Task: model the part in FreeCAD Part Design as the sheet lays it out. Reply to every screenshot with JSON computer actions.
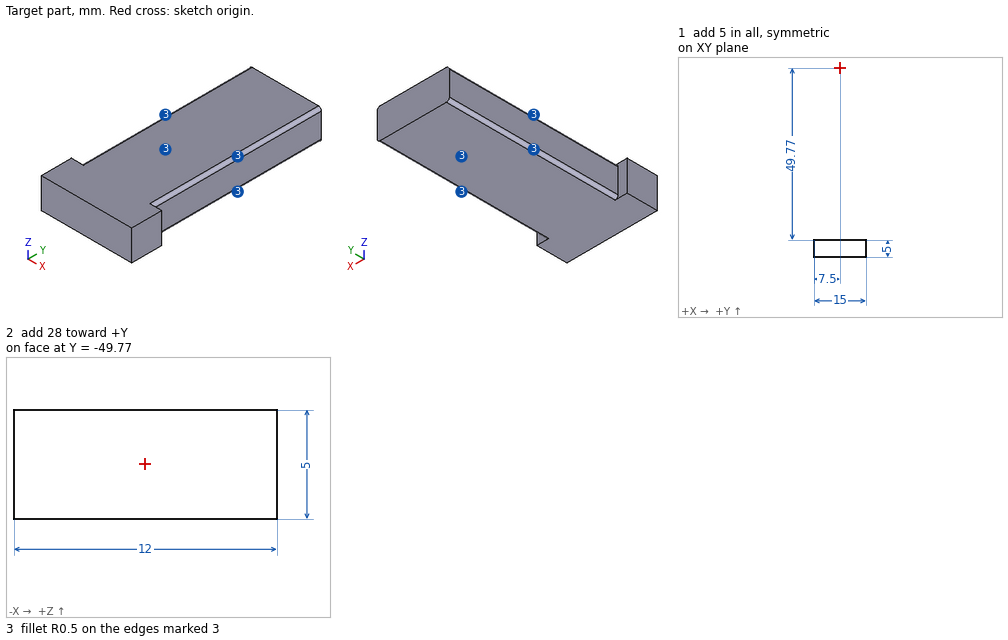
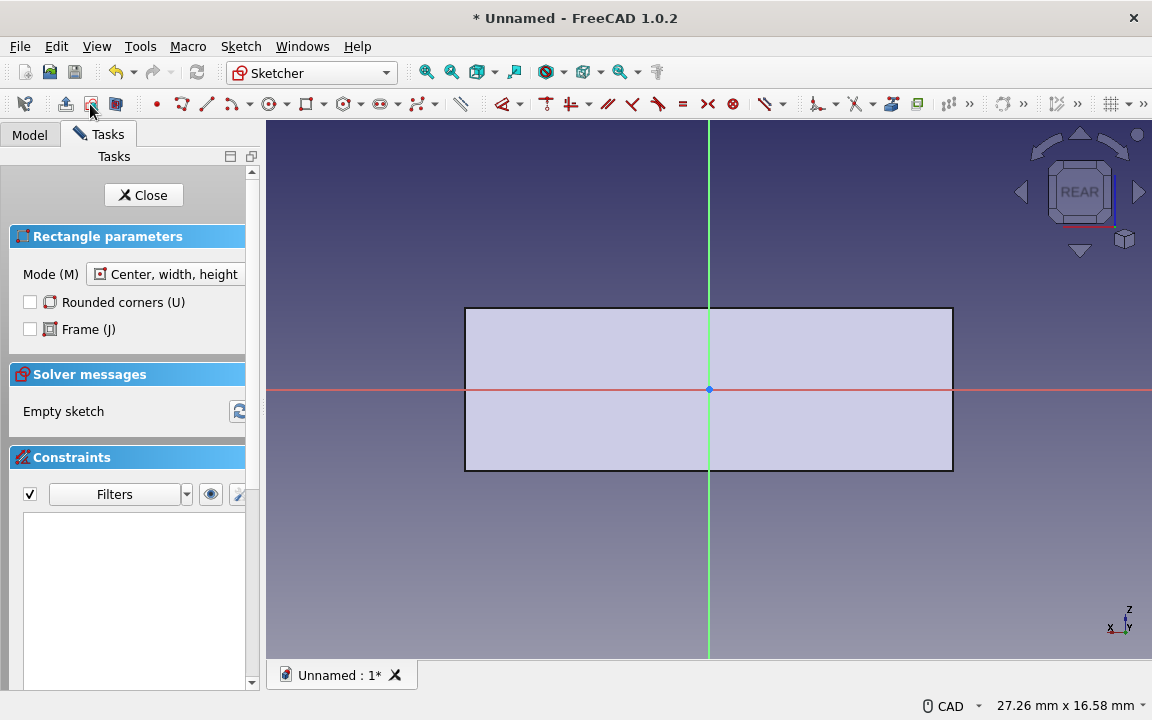
{"action": "left_click", "coordinate": [709, 390]}
{"action": "mouse_move", "coordinate": [904, 308]}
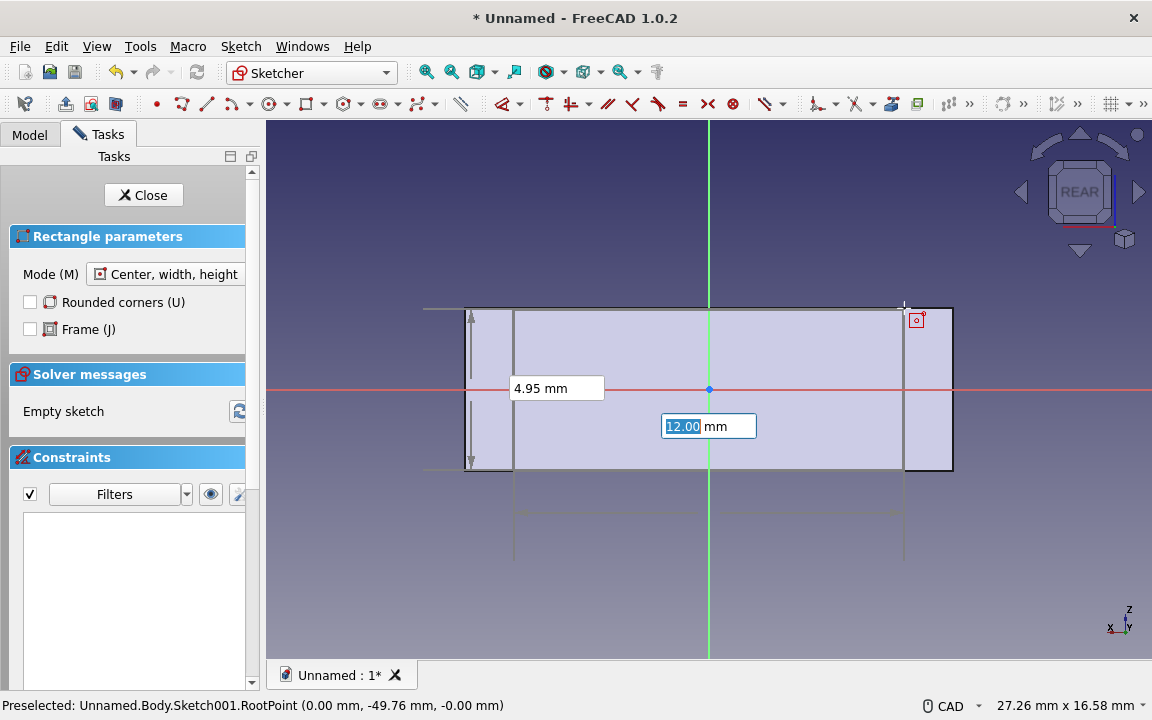
{"action": "type", "text": "12"}
{"action": "key", "text": "Tab"}
{"action": "type", "text": "5"}
{"action": "key", "text": "Return"}
{"action": "key", "text": "Escape"}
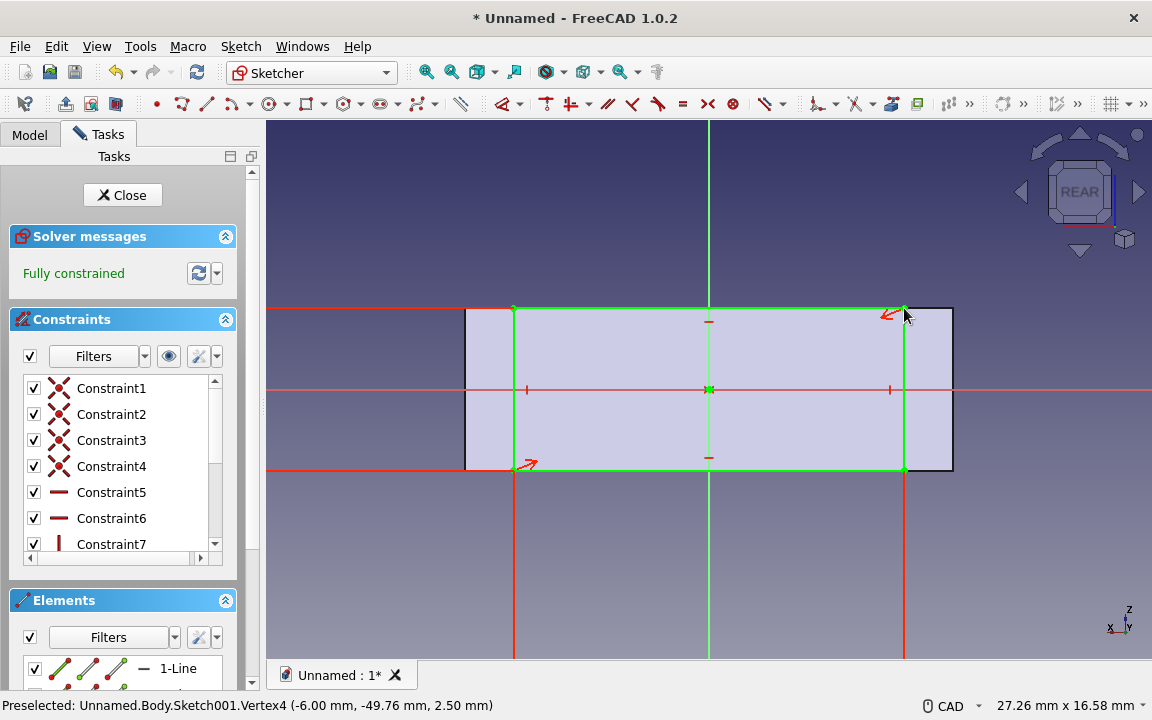
{"action": "left_click", "coordinate": [123, 195]}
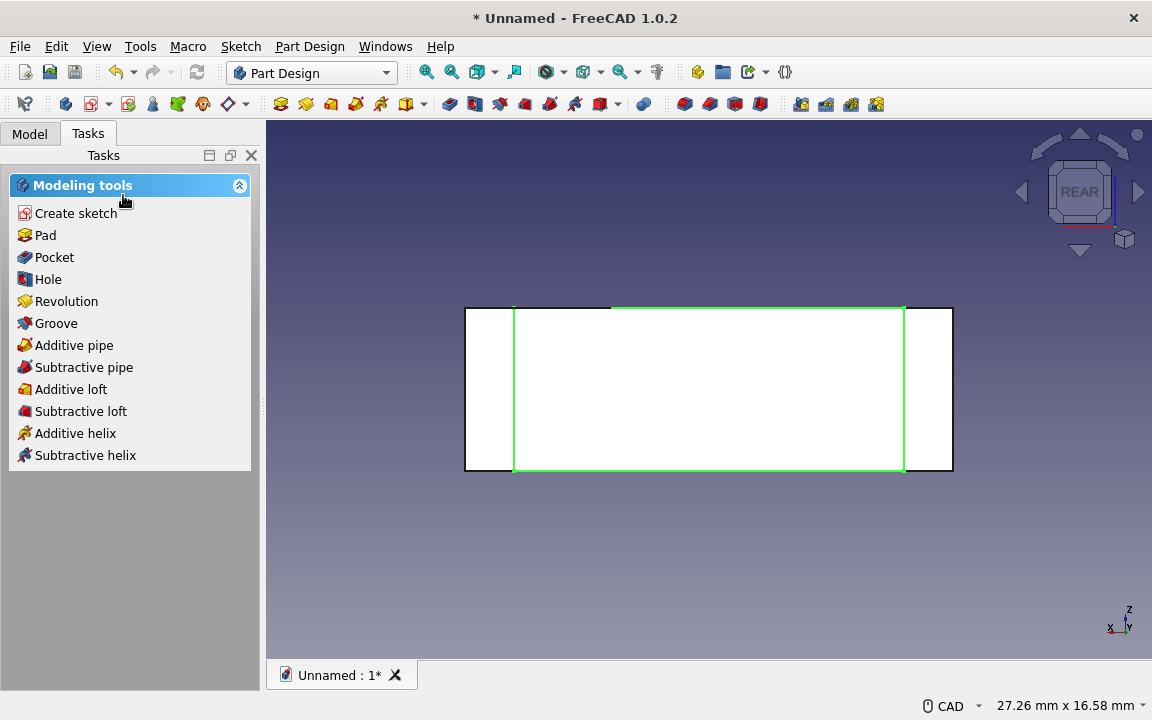
{"action": "left_click", "coordinate": [281, 104]}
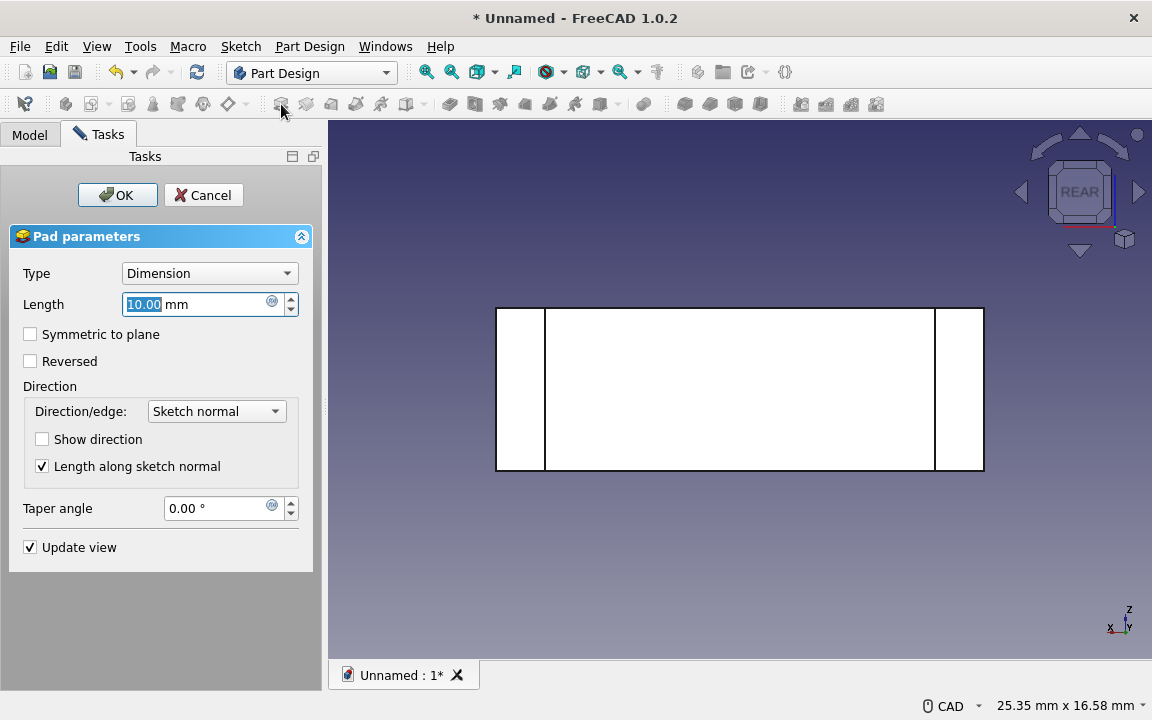
{"action": "type", "text": "28"}
{"action": "key", "text": "Tab"}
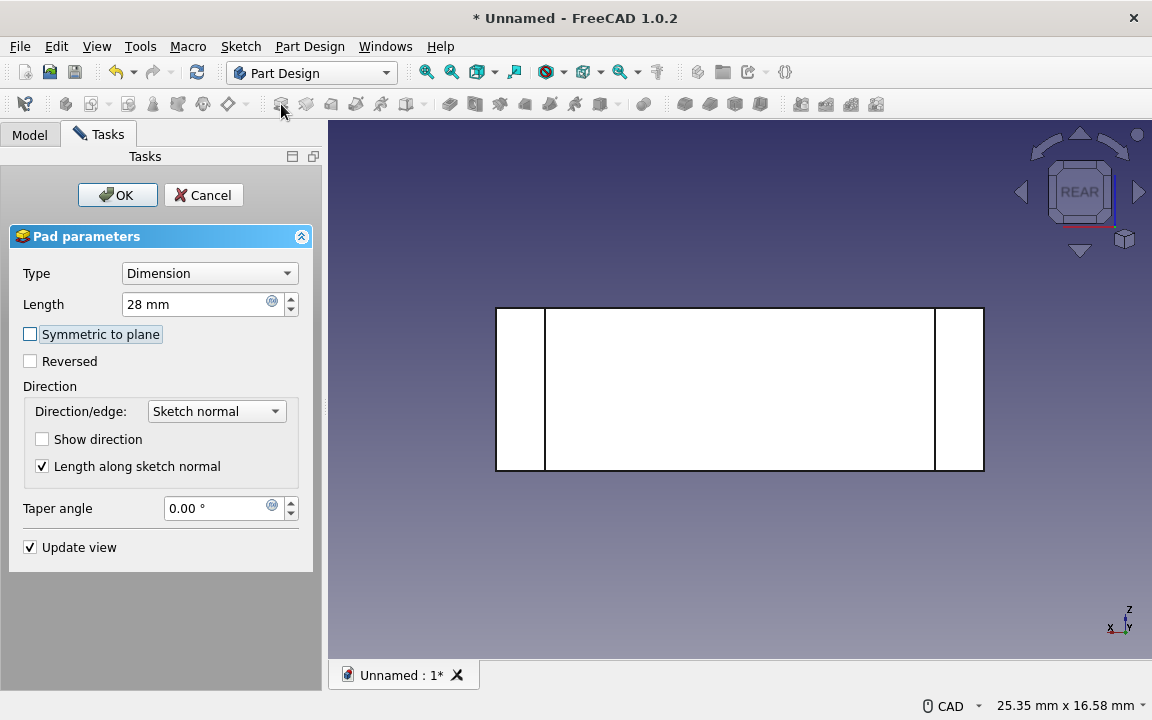
{"action": "left_click", "coordinate": [118, 195]}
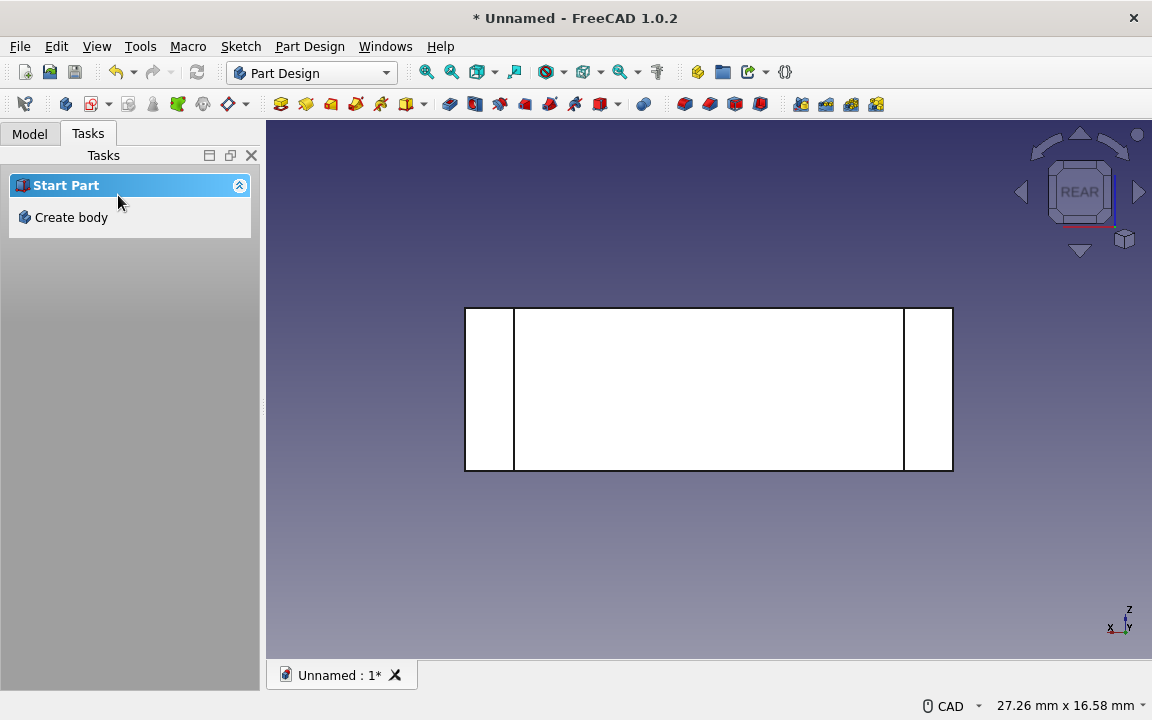
{"action": "key", "text": "0"}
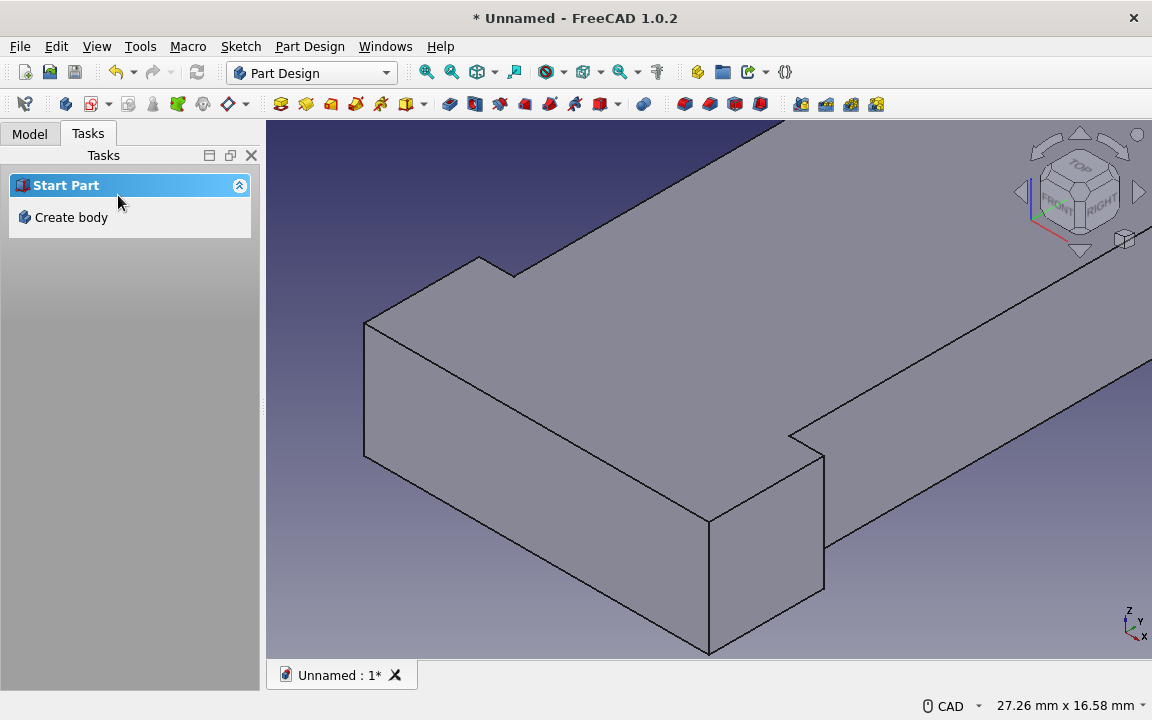
{"action": "left_click", "coordinate": [427, 72]}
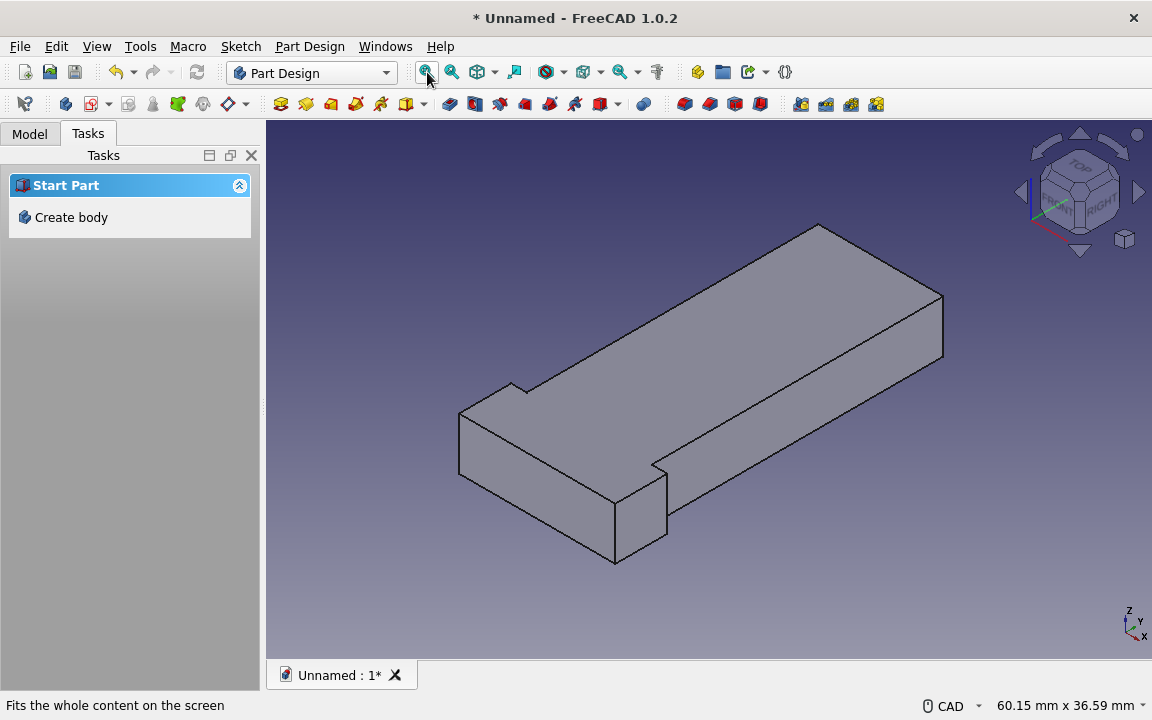
{"action": "left_click", "coordinate": [798, 379]}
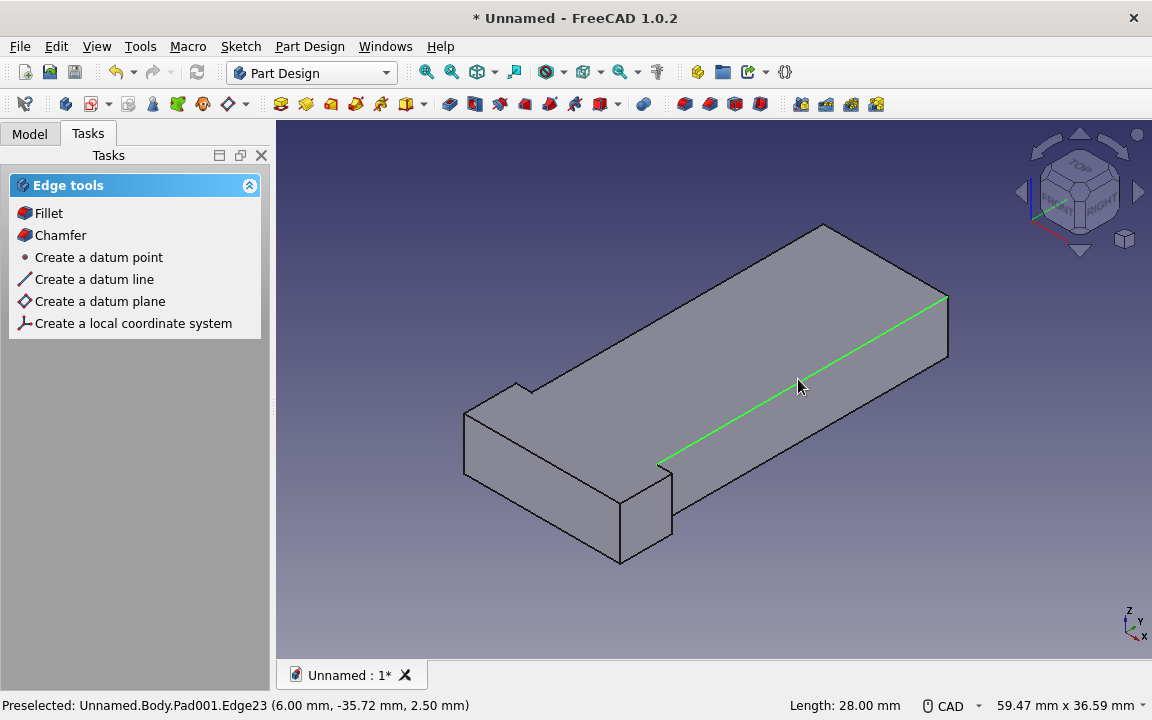
{"action": "key", "text": "2"}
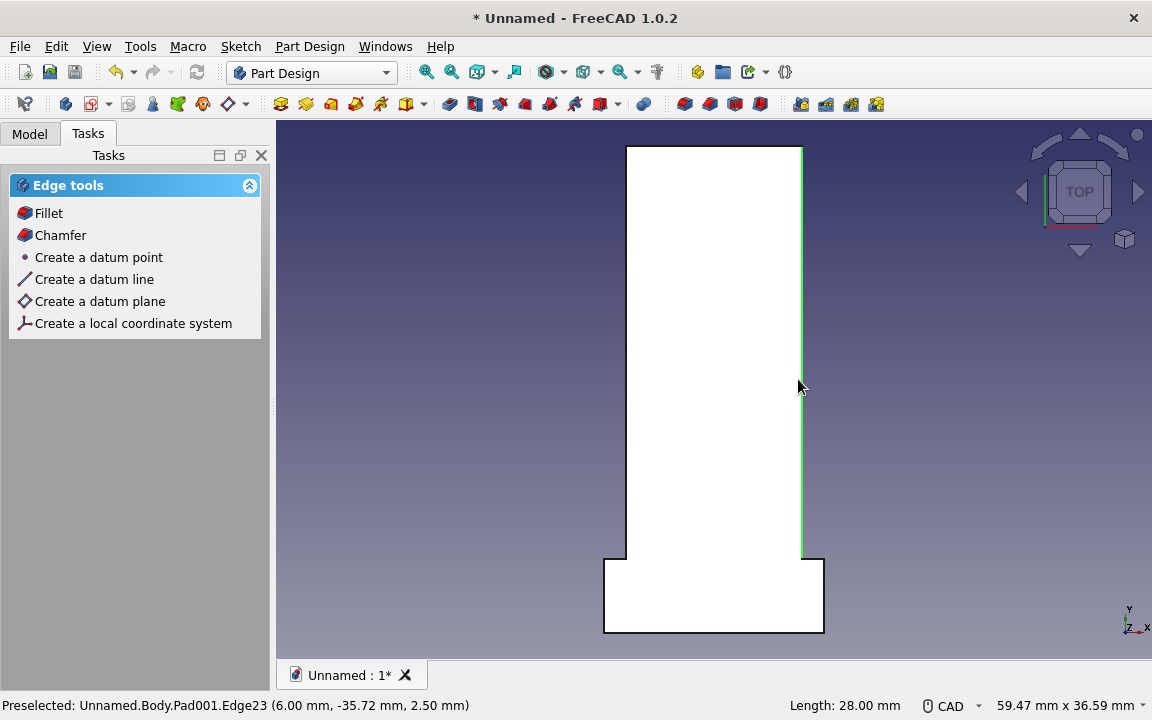
{"action": "left_click", "coordinate": [626, 352], "text": "ctrl"}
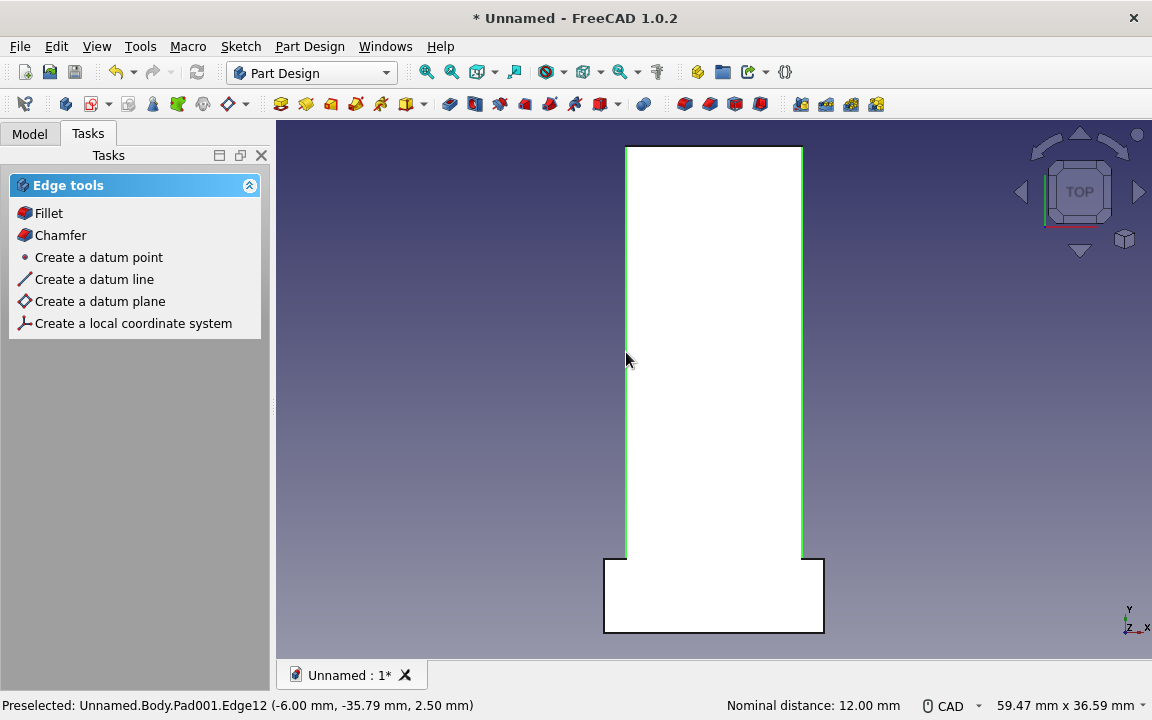
{"action": "key", "text": "1"}